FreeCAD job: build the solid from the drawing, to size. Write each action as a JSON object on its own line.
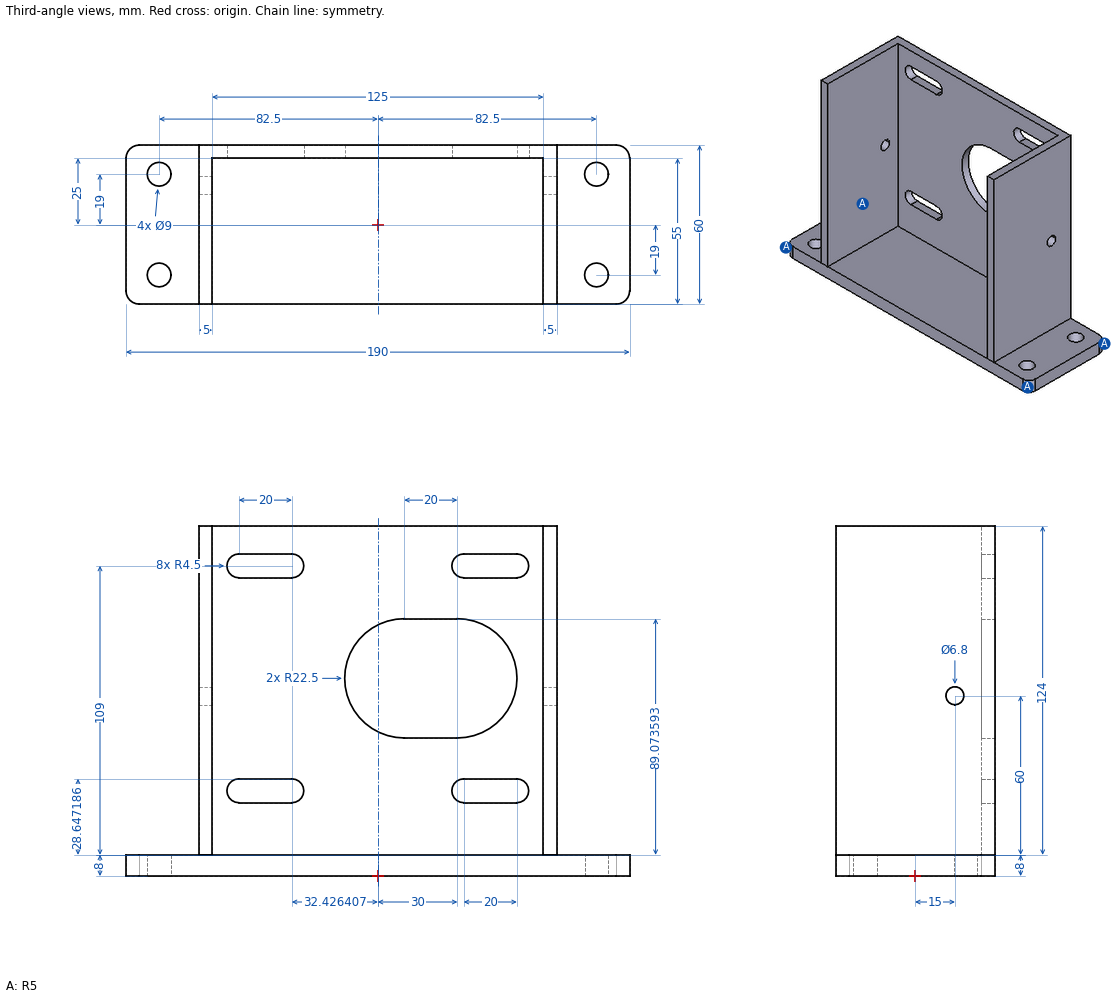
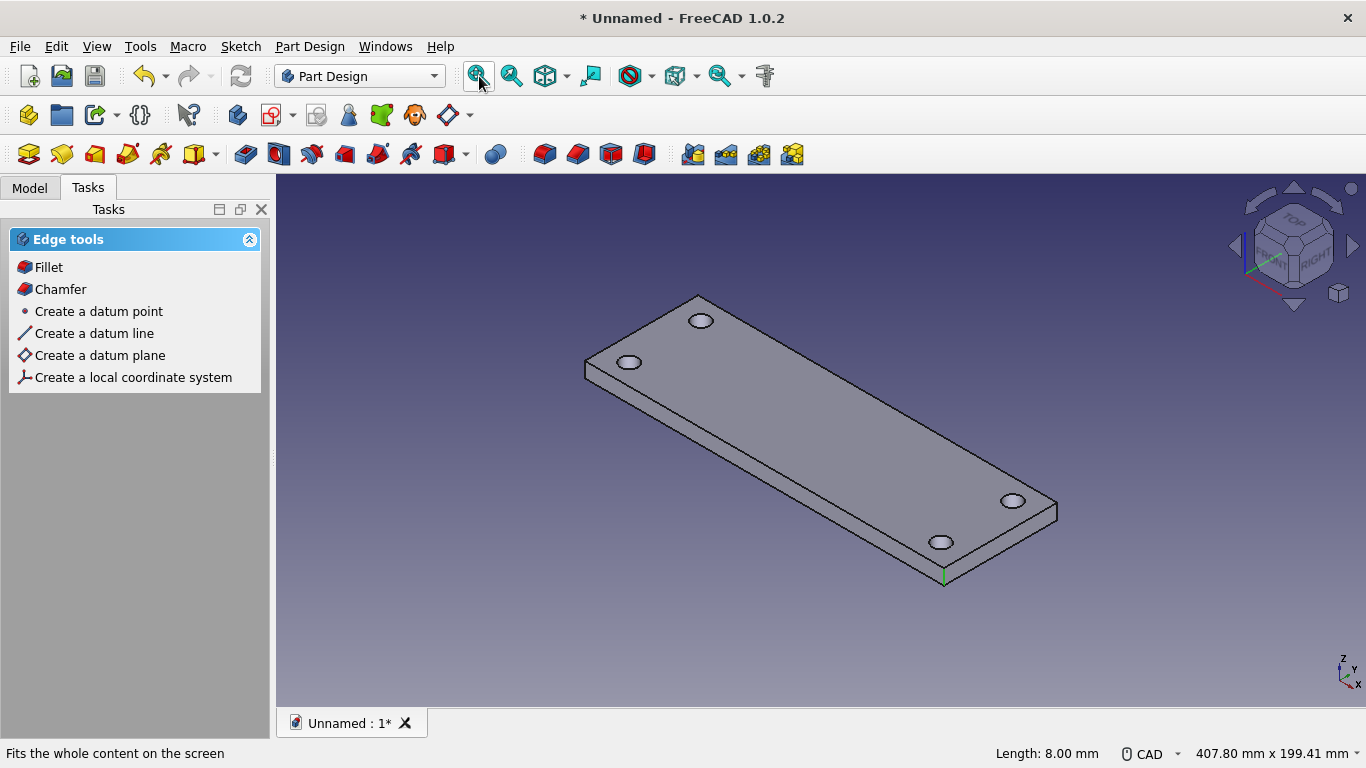
{"action": "key", "text": "2"}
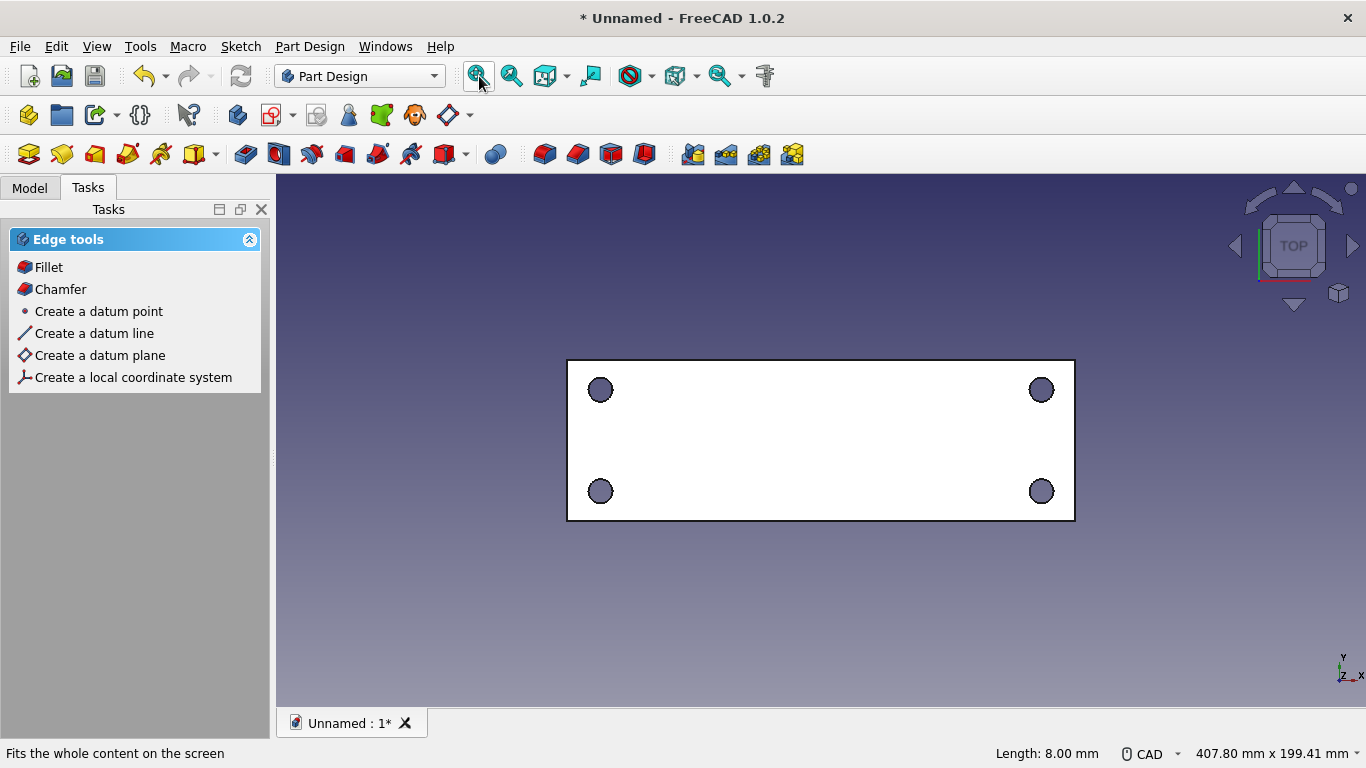
{"action": "scroll", "coordinate": [567, 520], "scroll_direction": "up", "scroll_amount": 4}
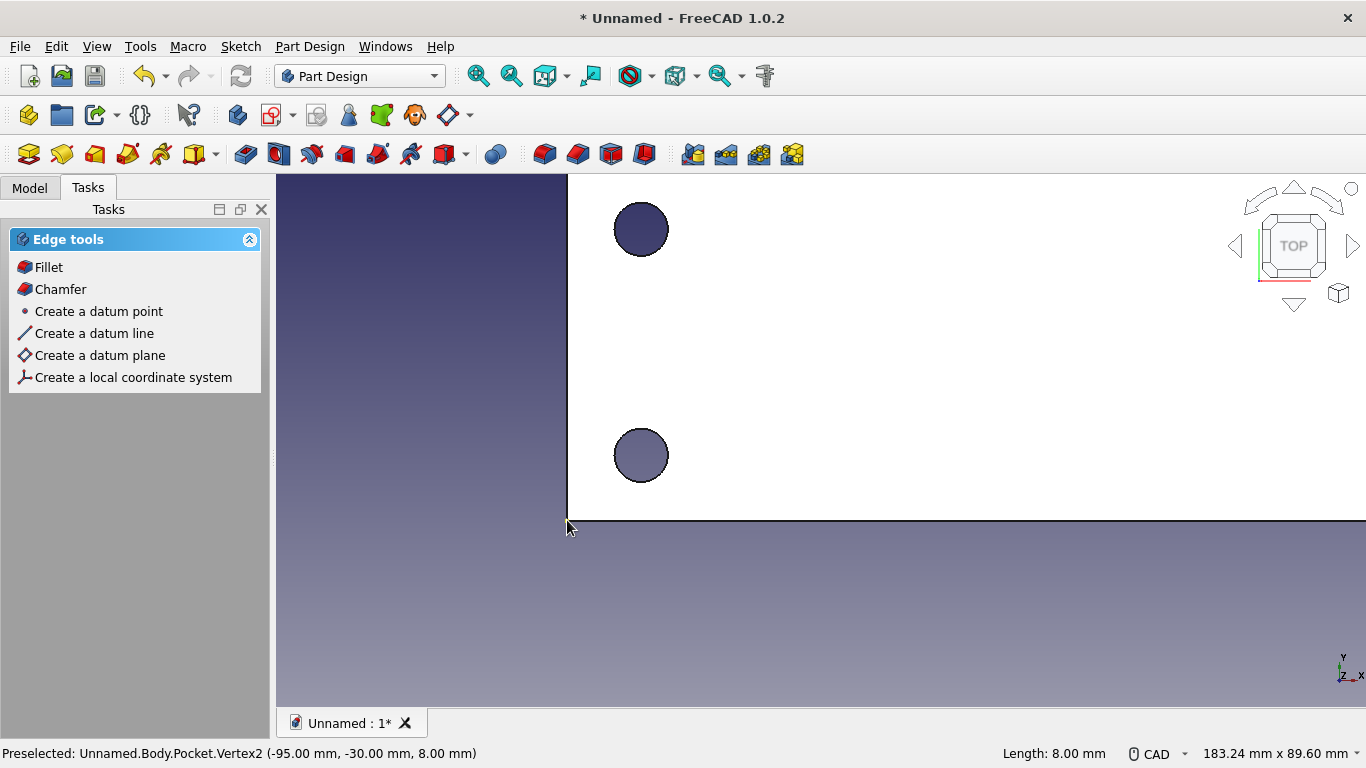
{"action": "key", "text": "v f"}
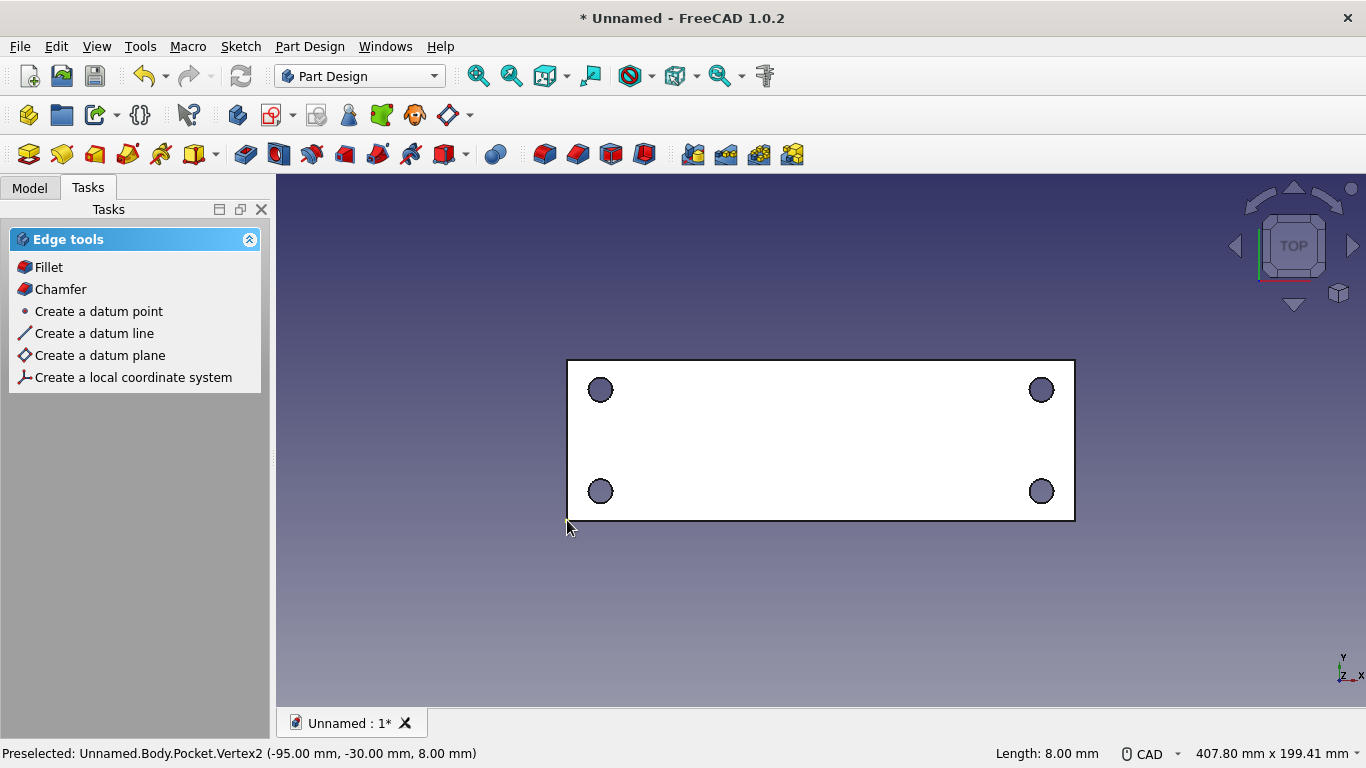
{"action": "key", "text": "1"}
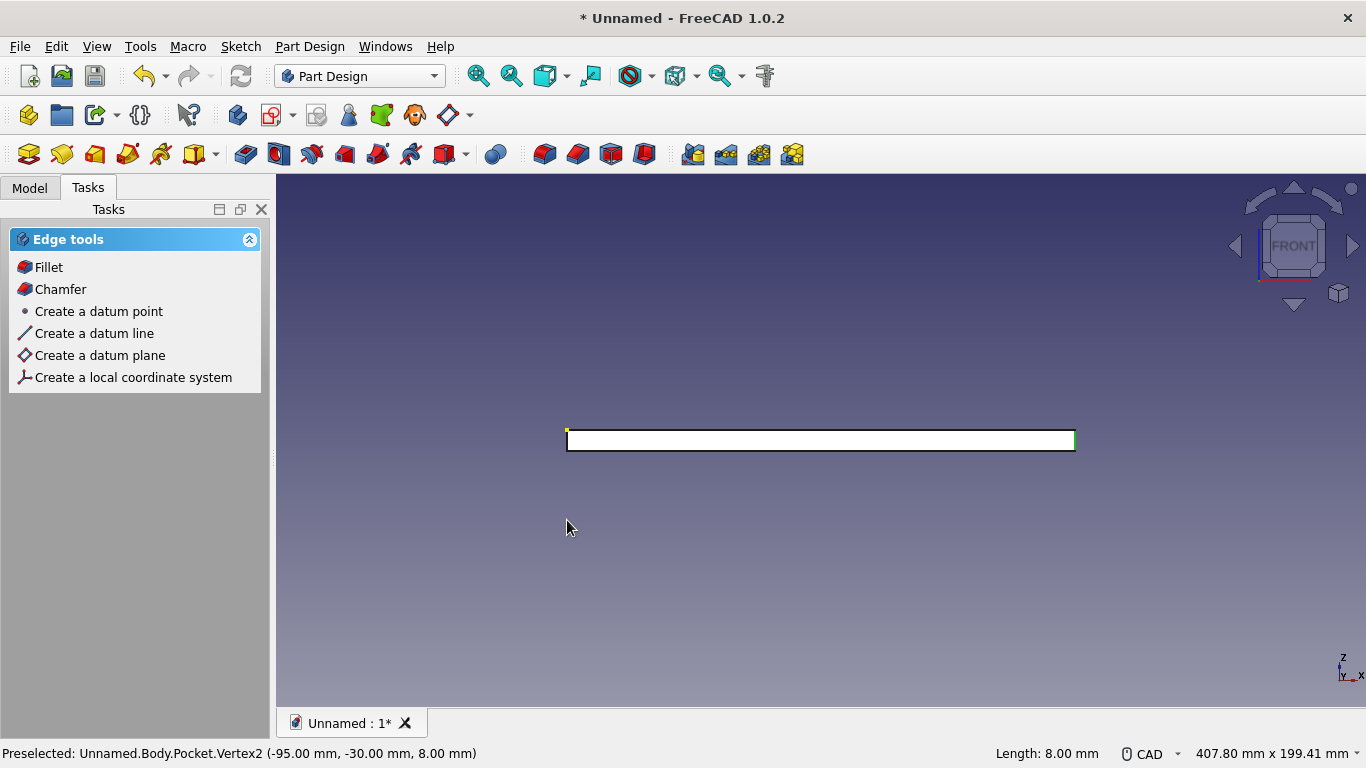
{"action": "left_click", "coordinate": [567, 439], "text": "ctrl"}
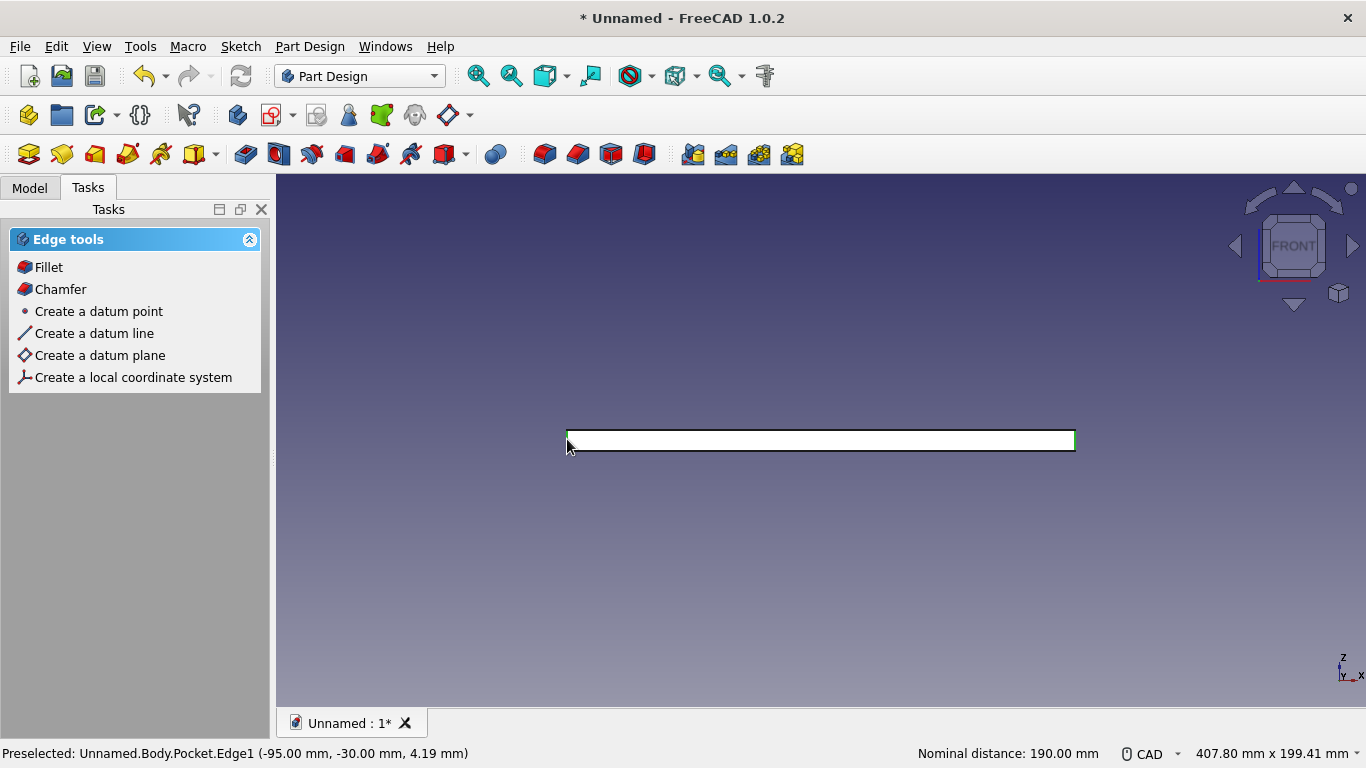
{"action": "scroll", "coordinate": [567, 439], "scroll_direction": "up", "scroll_amount": 4}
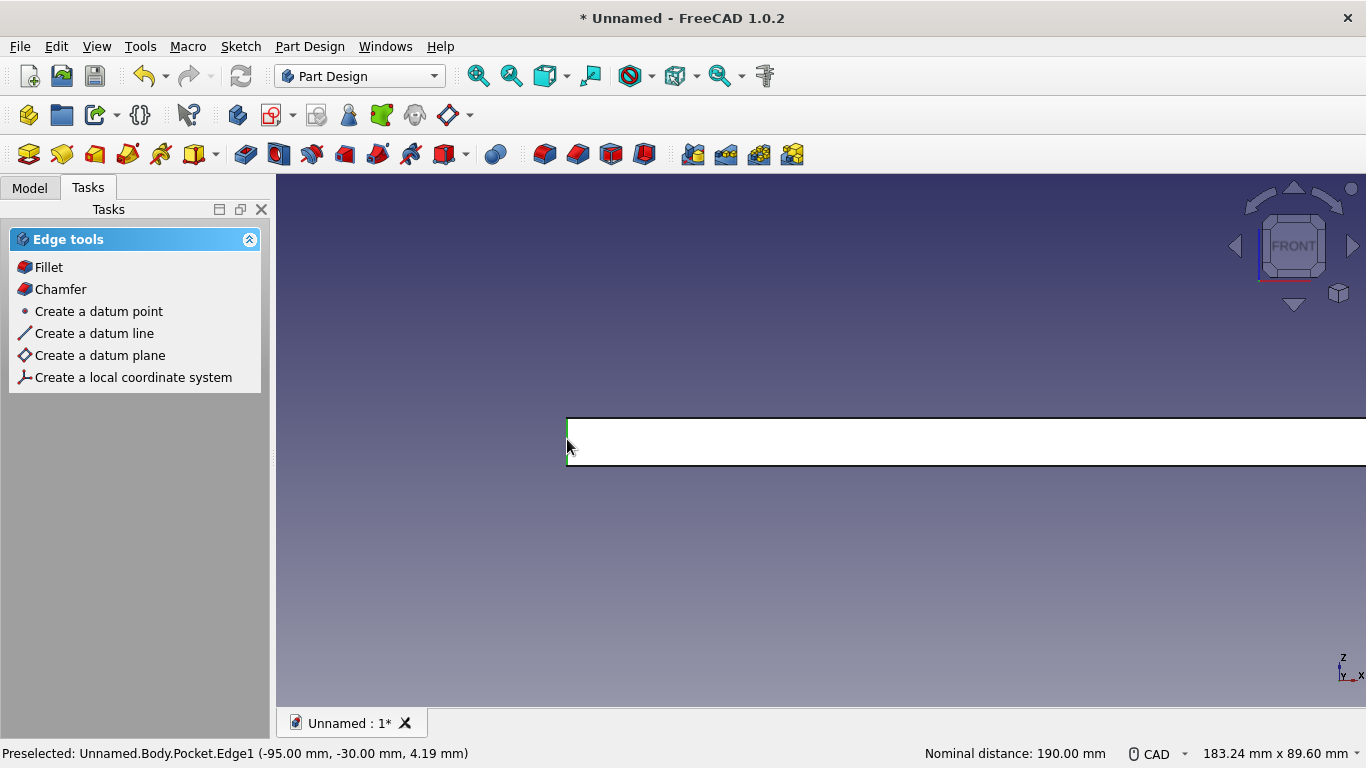
{"action": "left_click", "coordinate": [479, 76]}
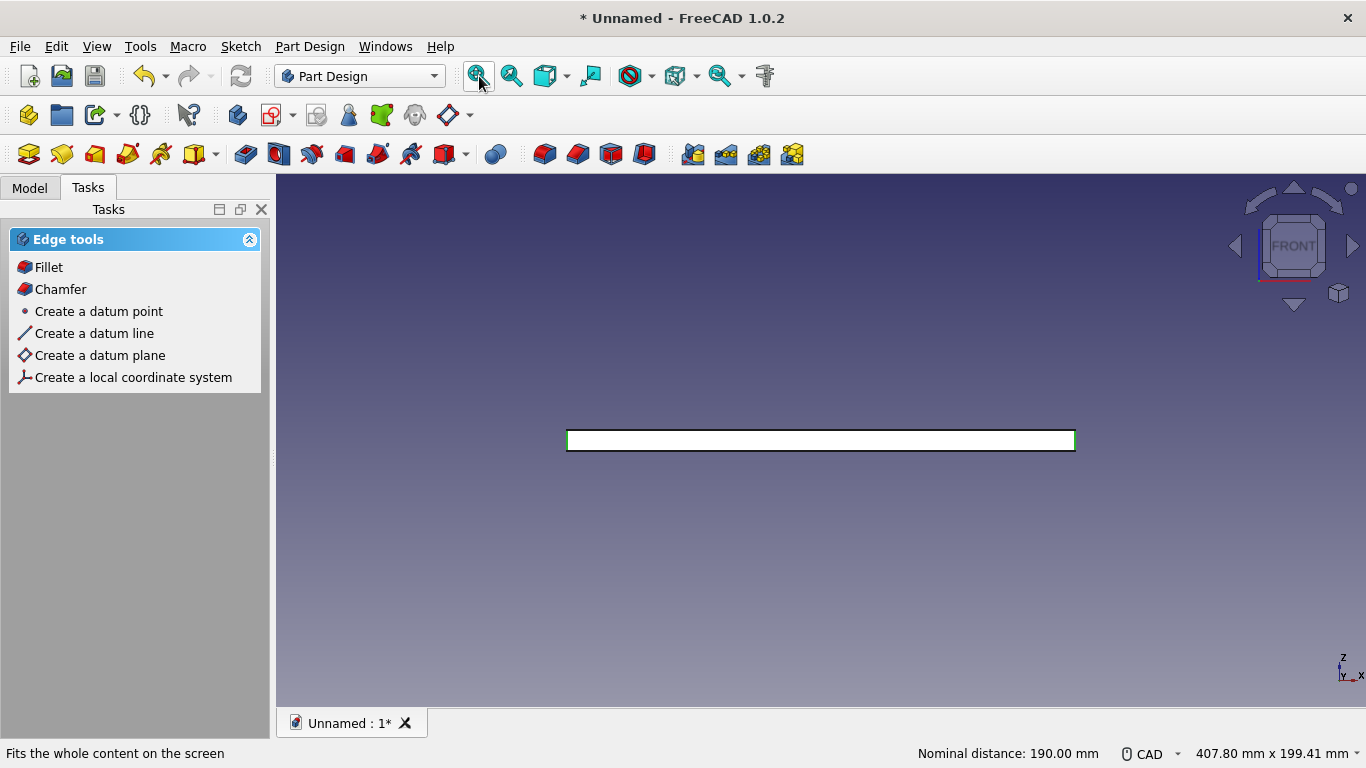
{"action": "key", "text": "3"}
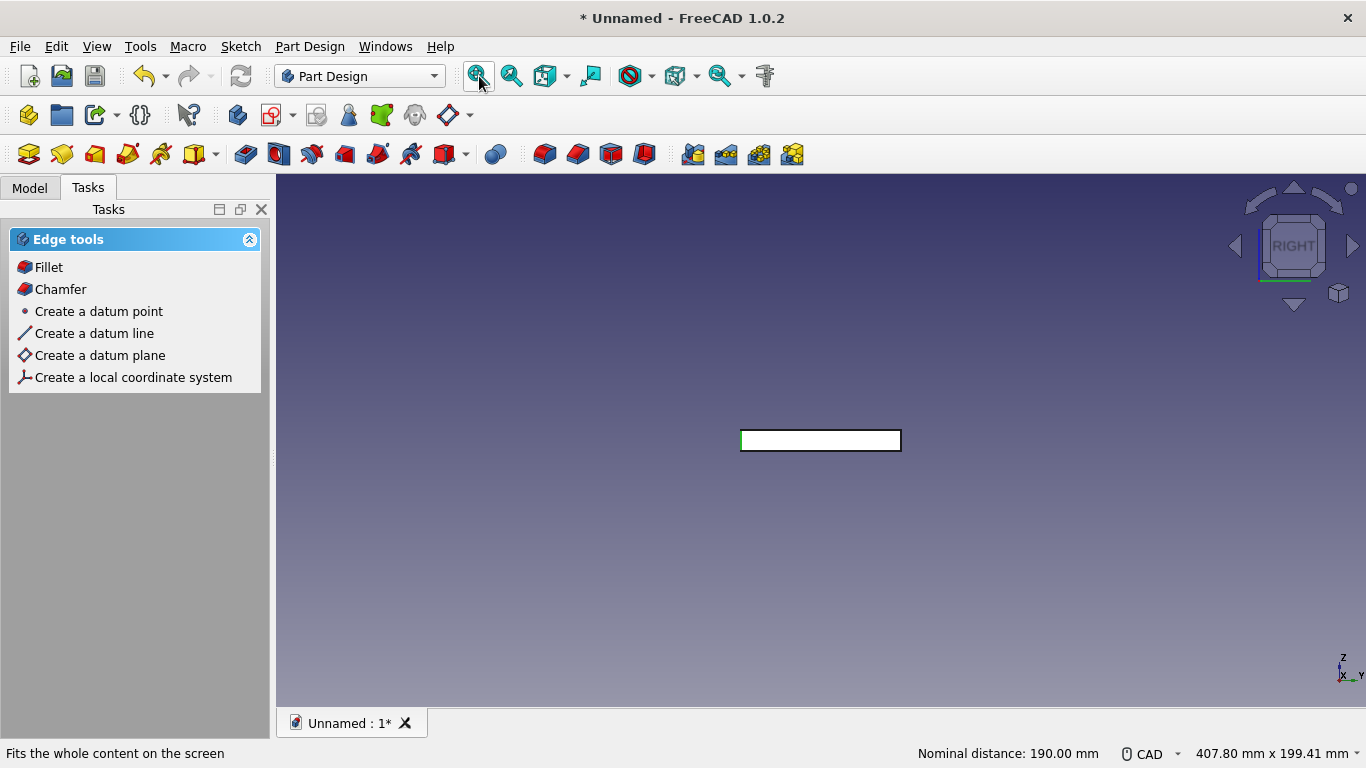
{"action": "left_click", "coordinate": [479, 76]}